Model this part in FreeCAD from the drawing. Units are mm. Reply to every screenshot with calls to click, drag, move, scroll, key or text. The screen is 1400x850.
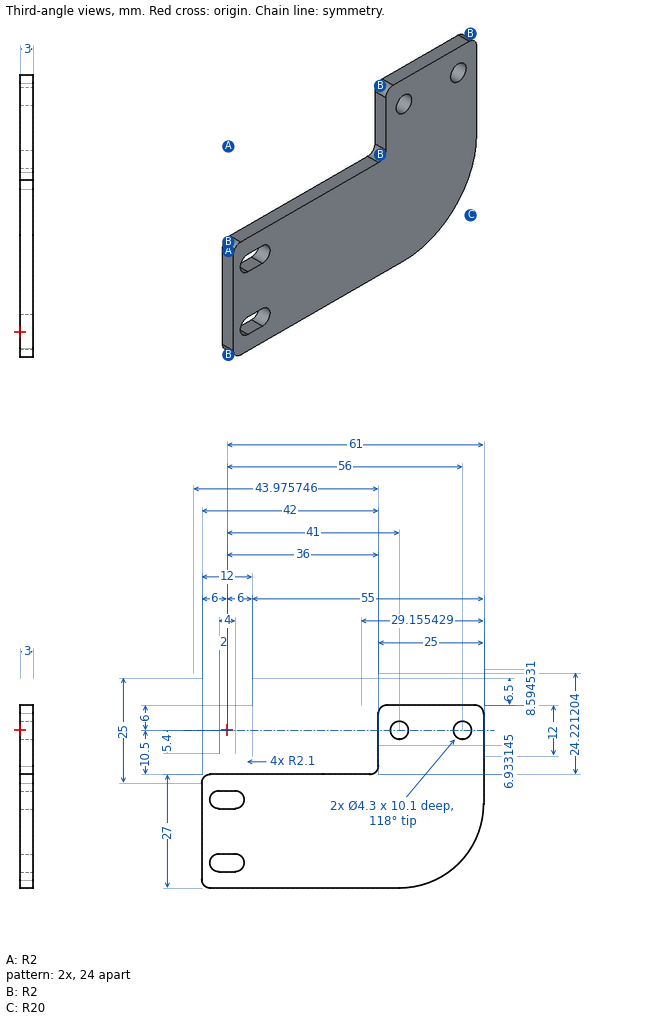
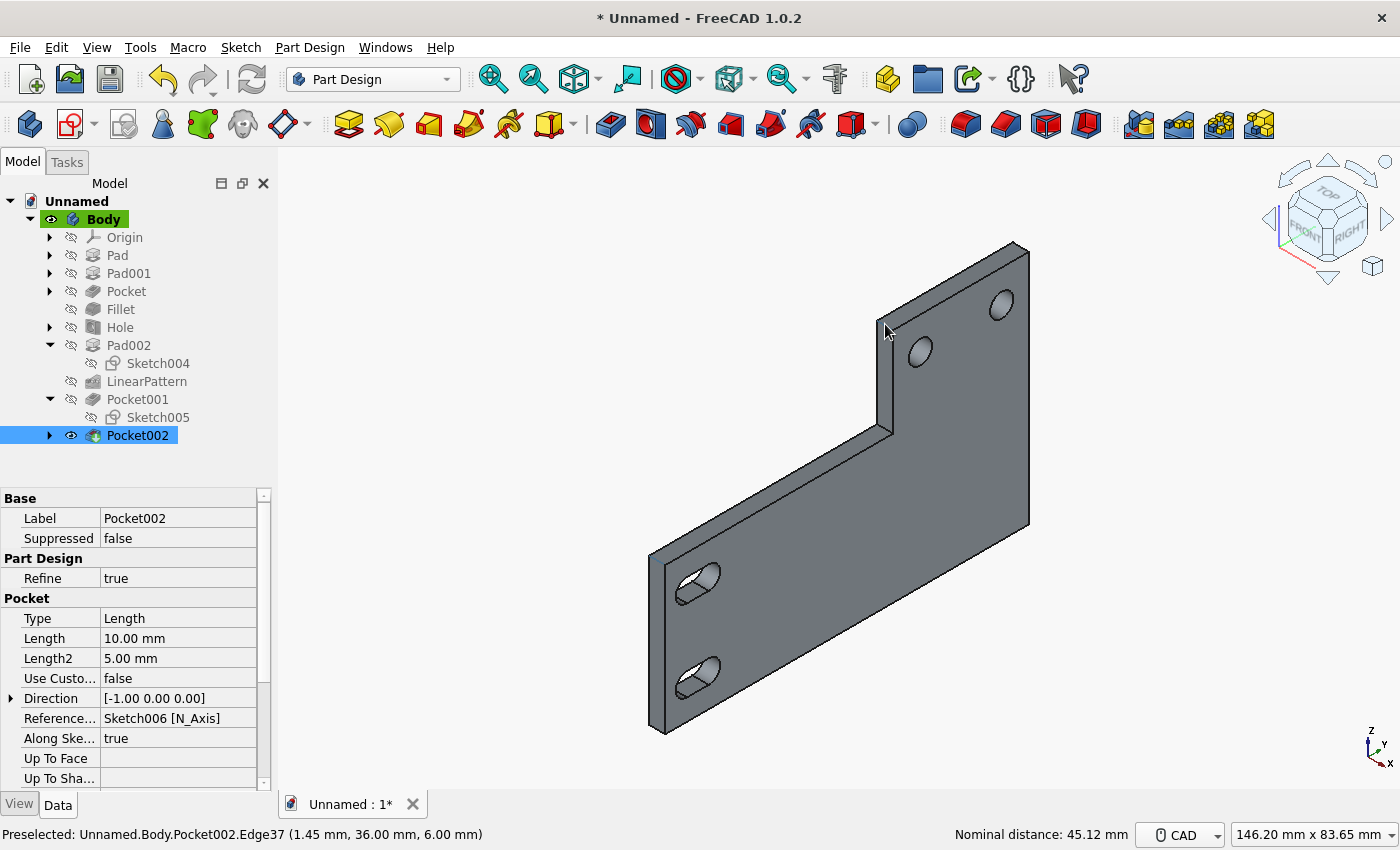
key(2)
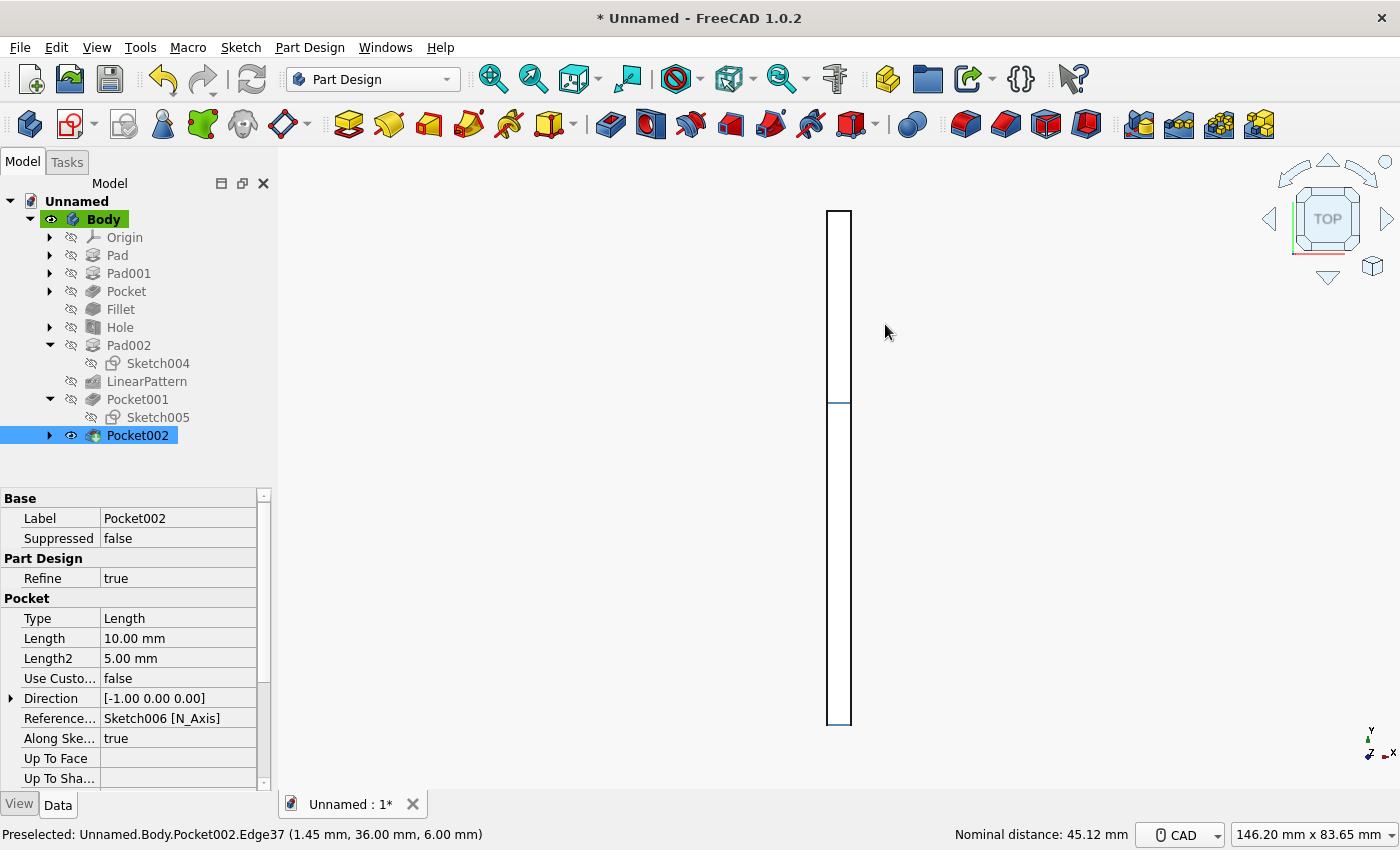
click(839, 210, ctrl)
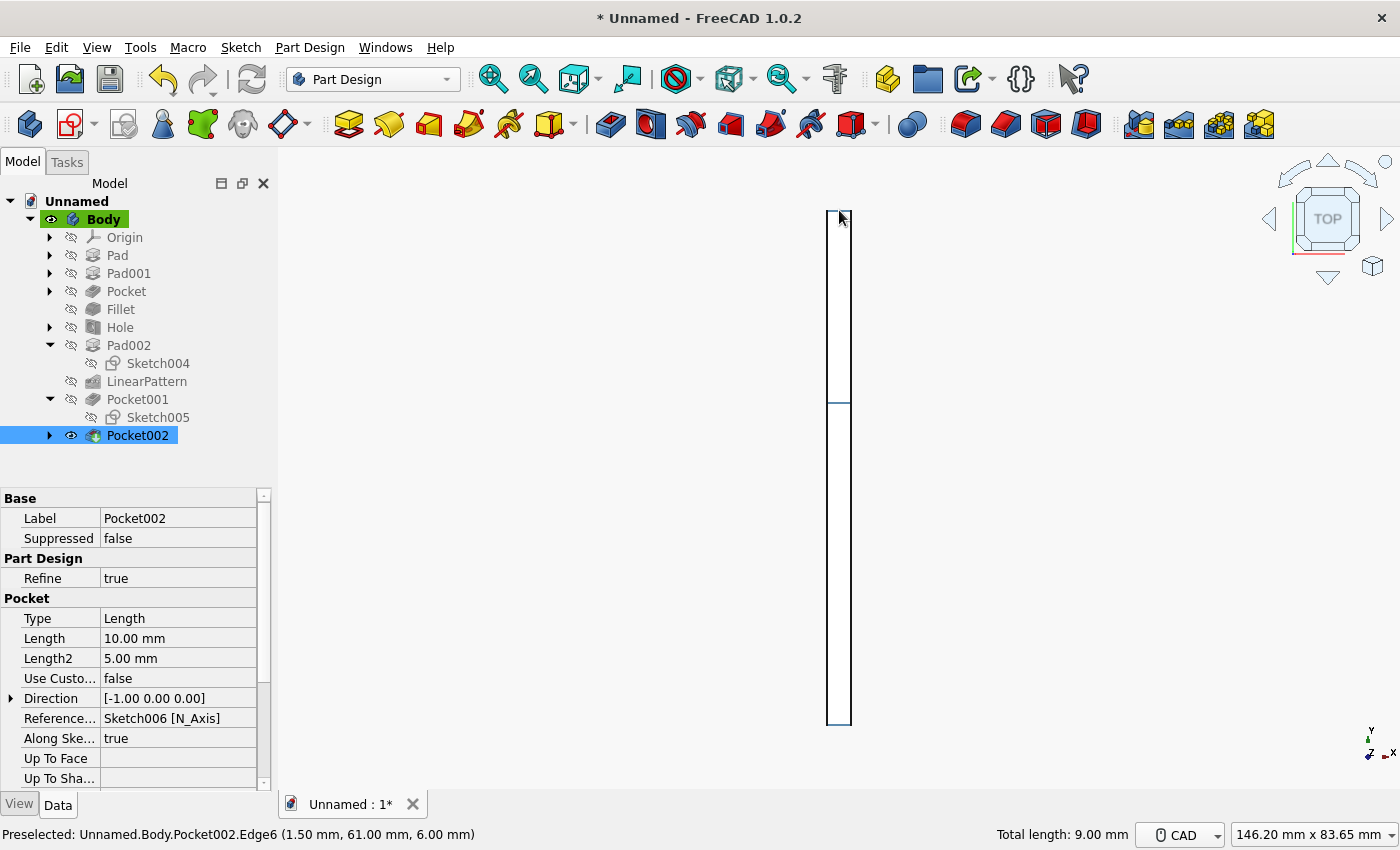
key(1)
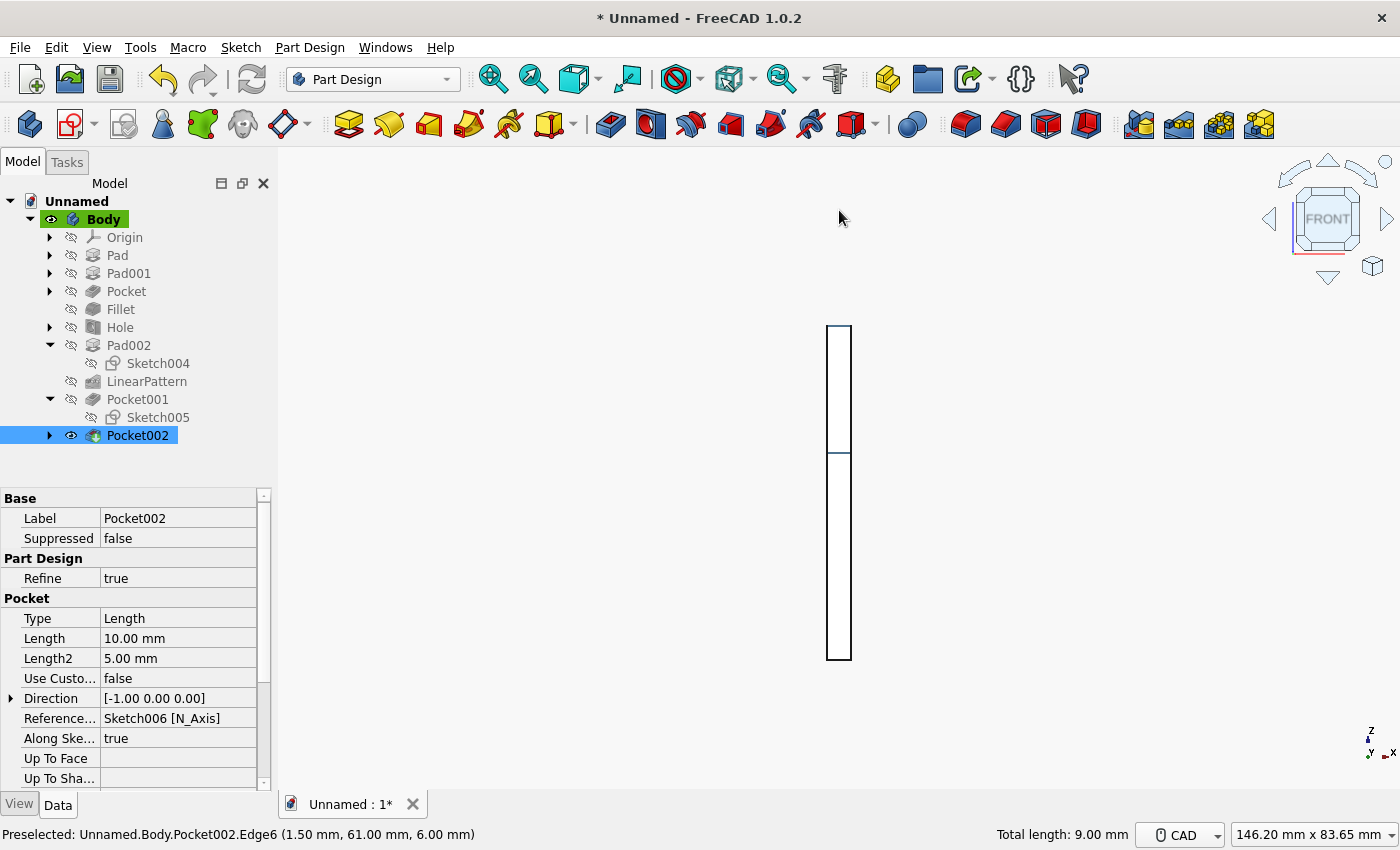
click(839, 659, ctrl)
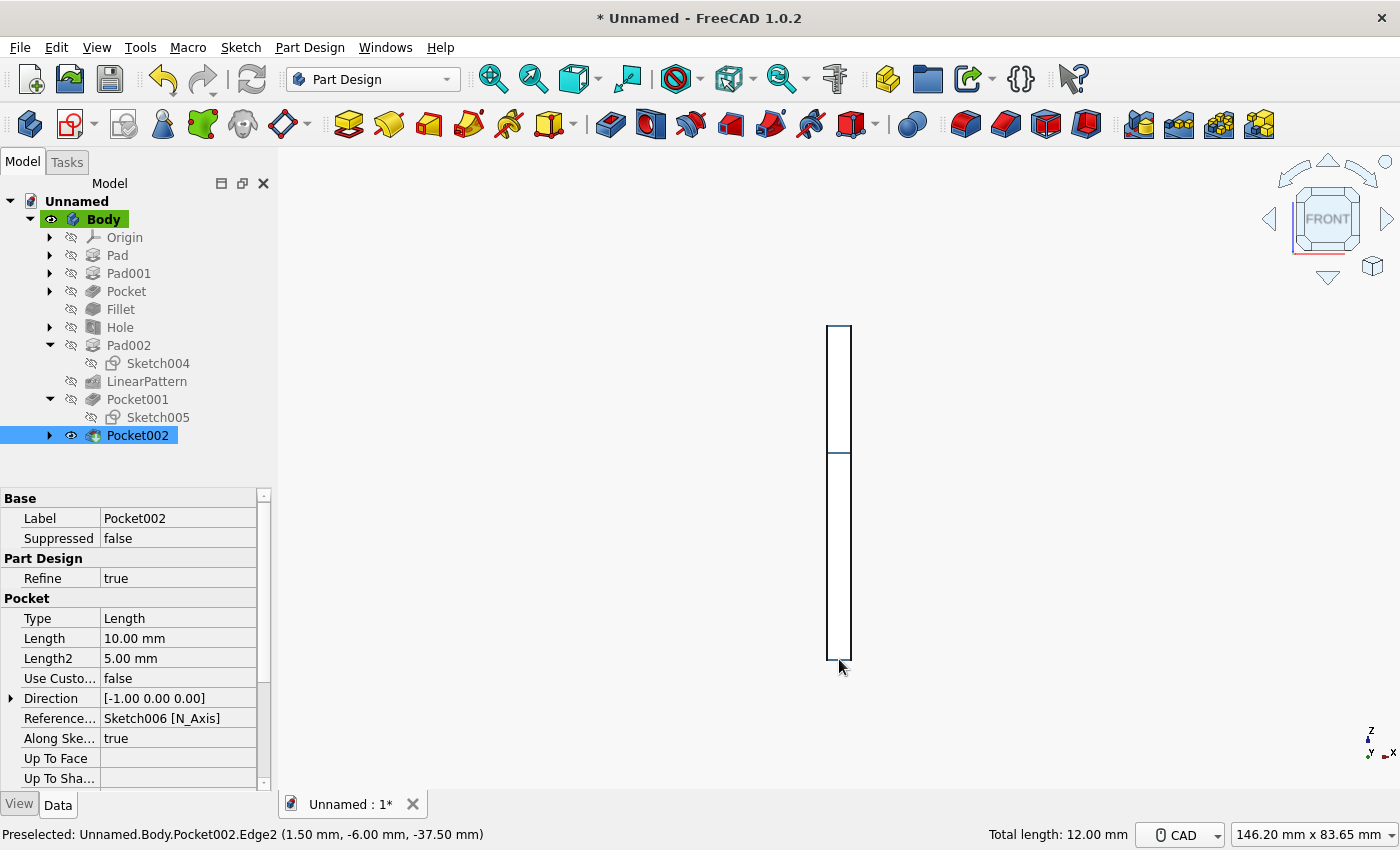
key(3)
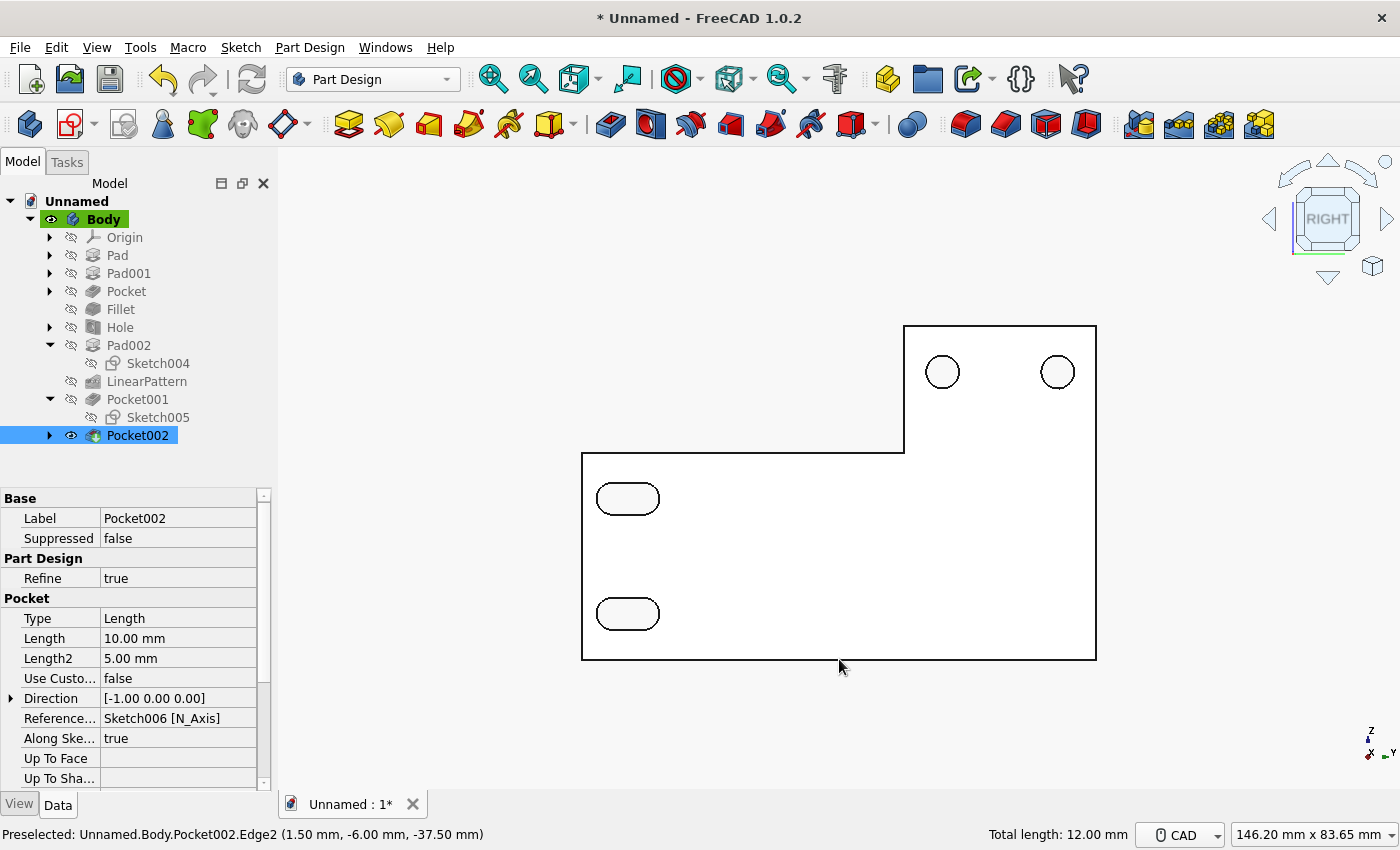
key(5)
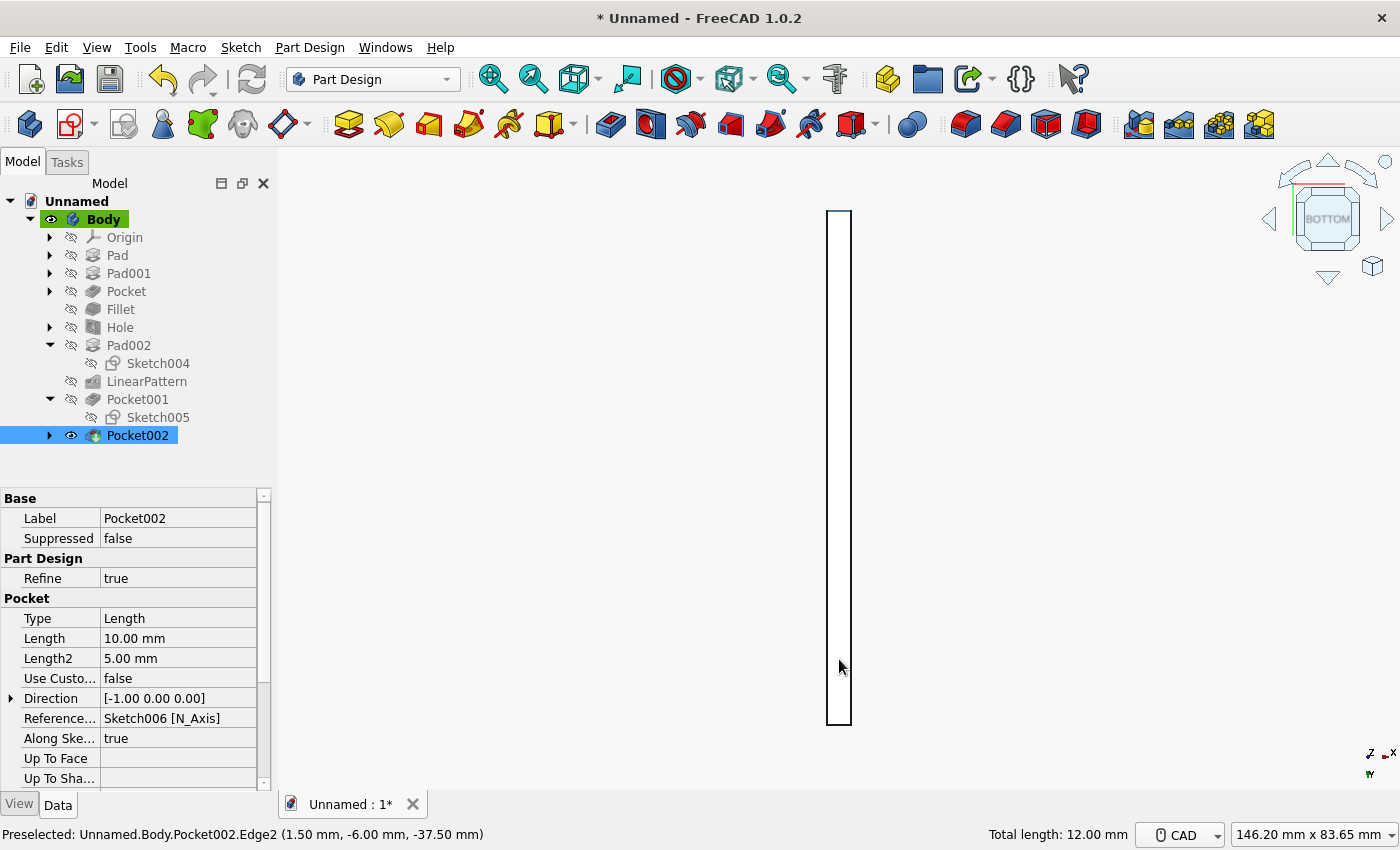
key(4)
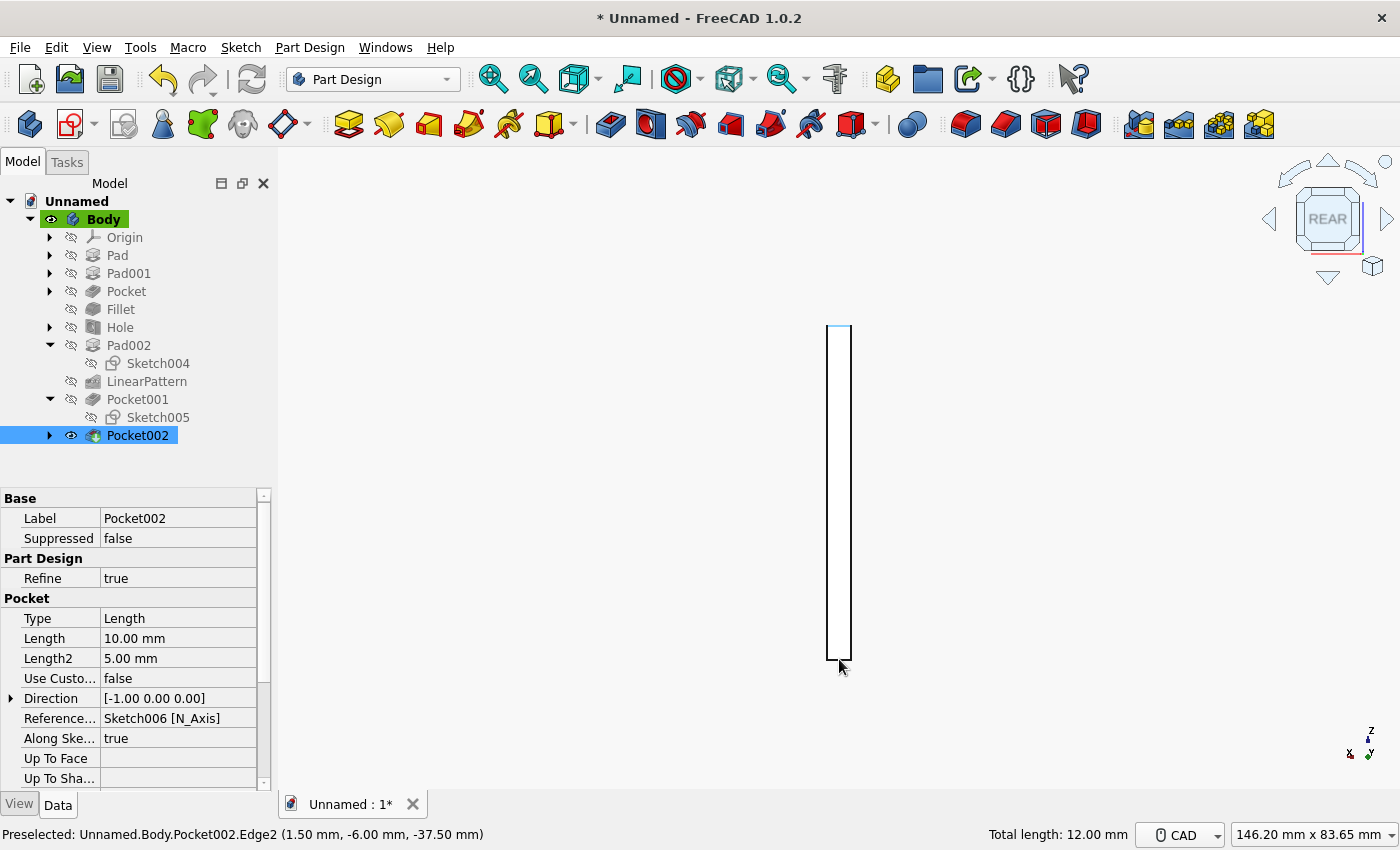
key(6)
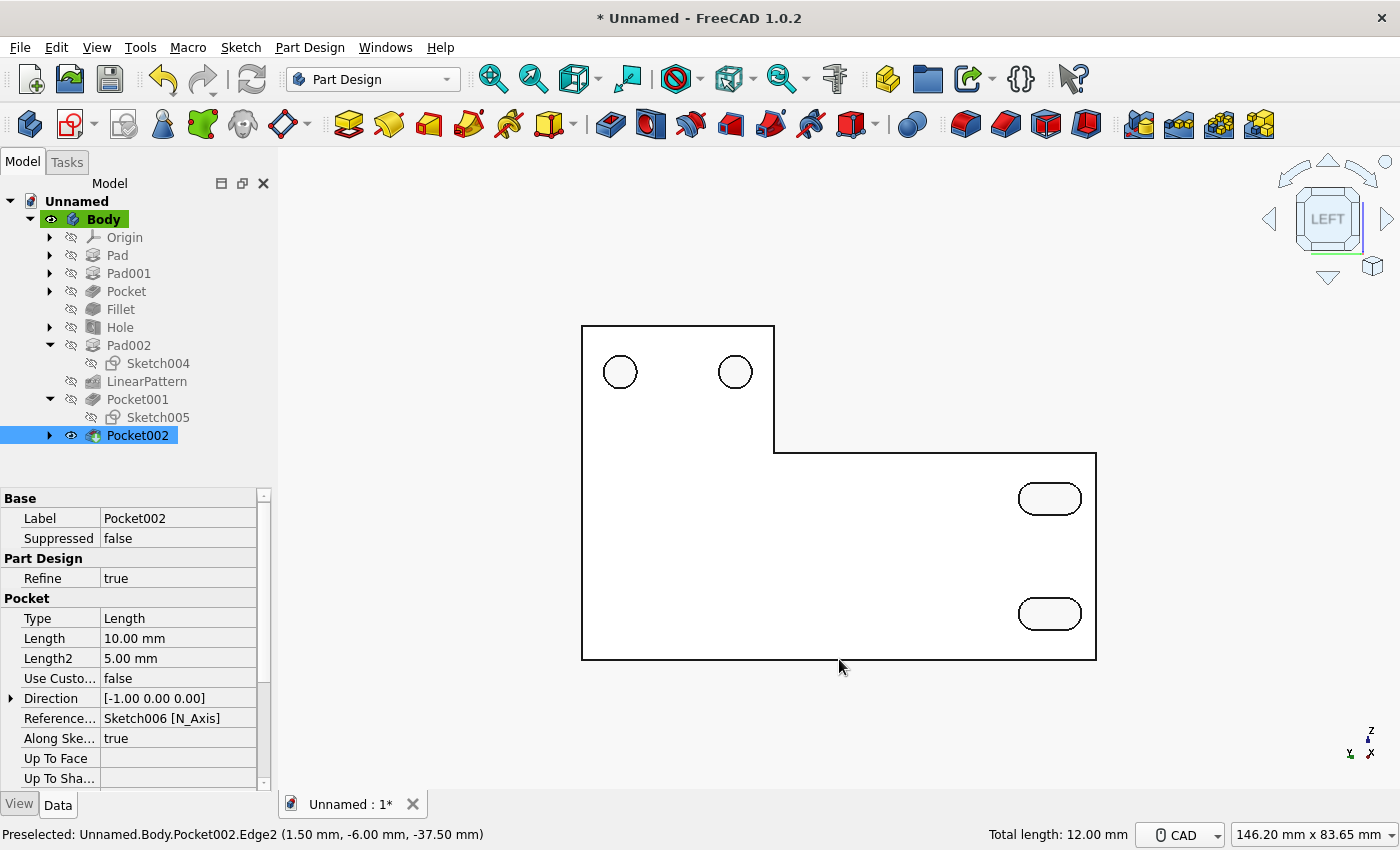
key(v)
key(3)